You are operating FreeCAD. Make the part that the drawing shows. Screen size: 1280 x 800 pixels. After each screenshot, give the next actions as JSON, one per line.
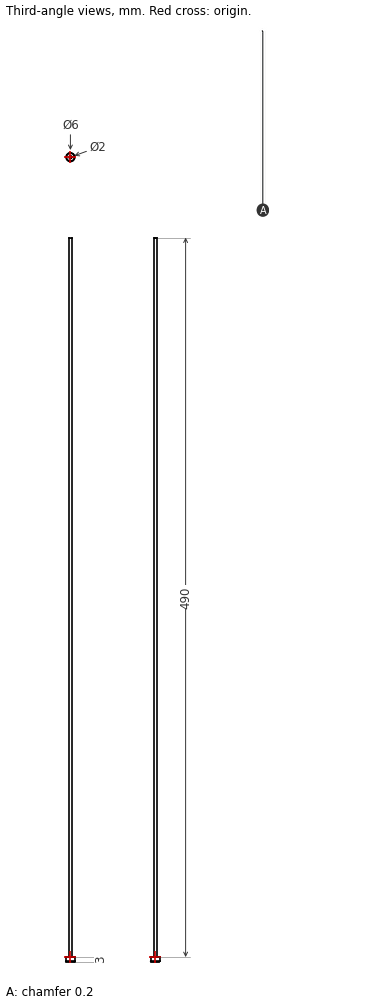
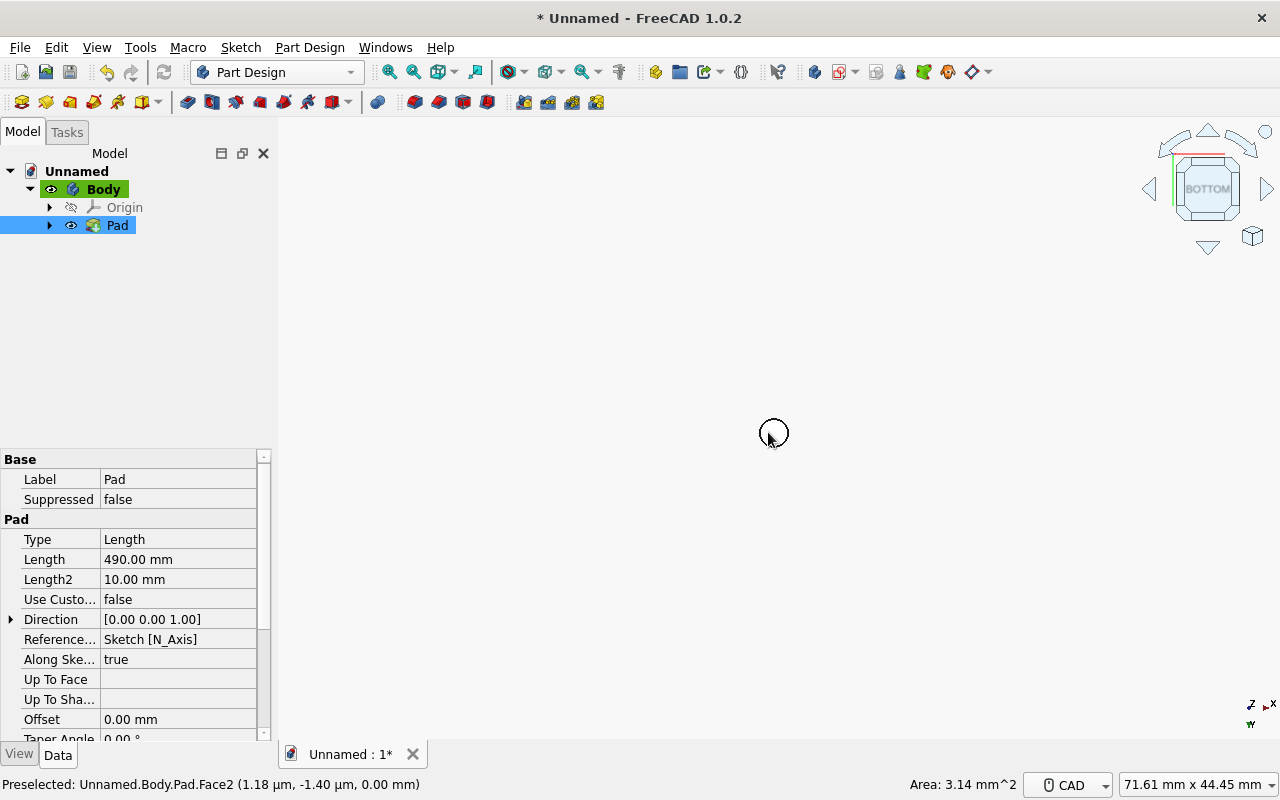
{"action": "left_click", "coordinate": [840, 72]}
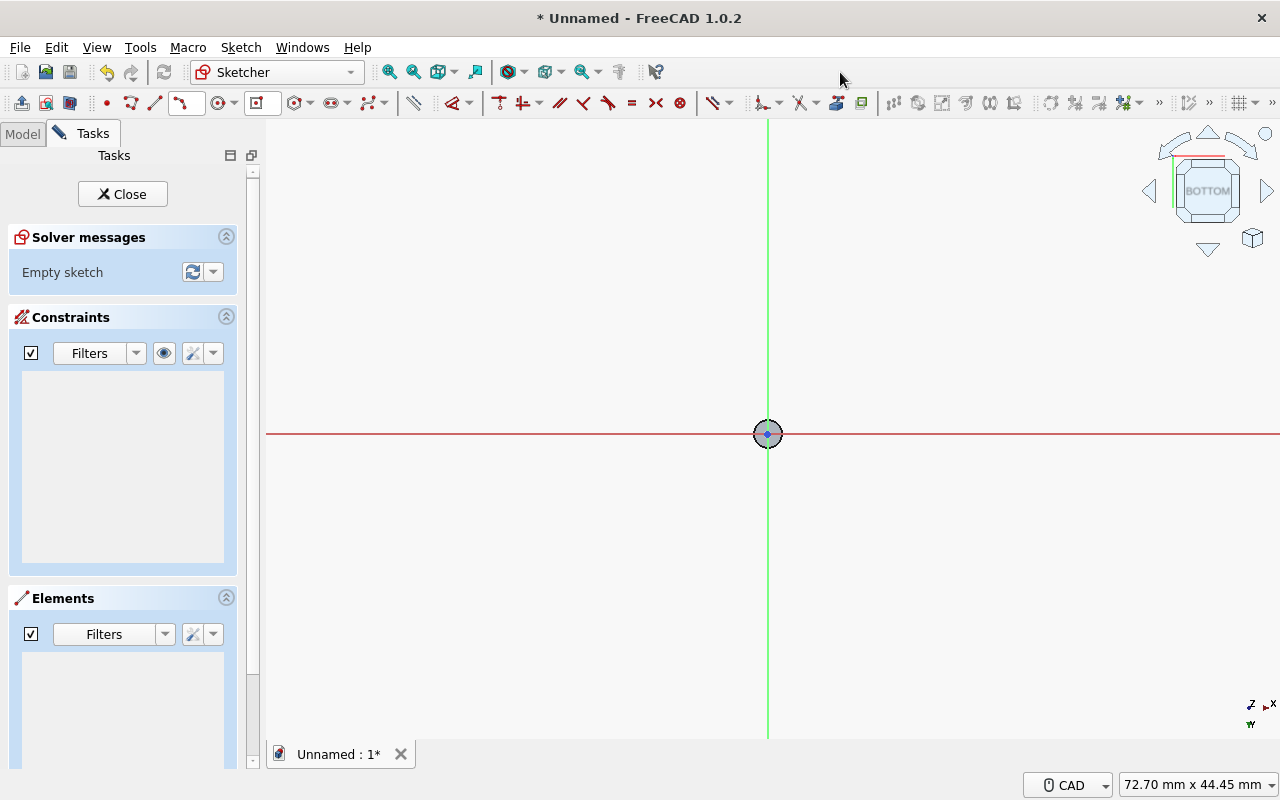
{"action": "scroll", "coordinate": [784, 435], "scroll_direction": "up", "scroll_amount": 8}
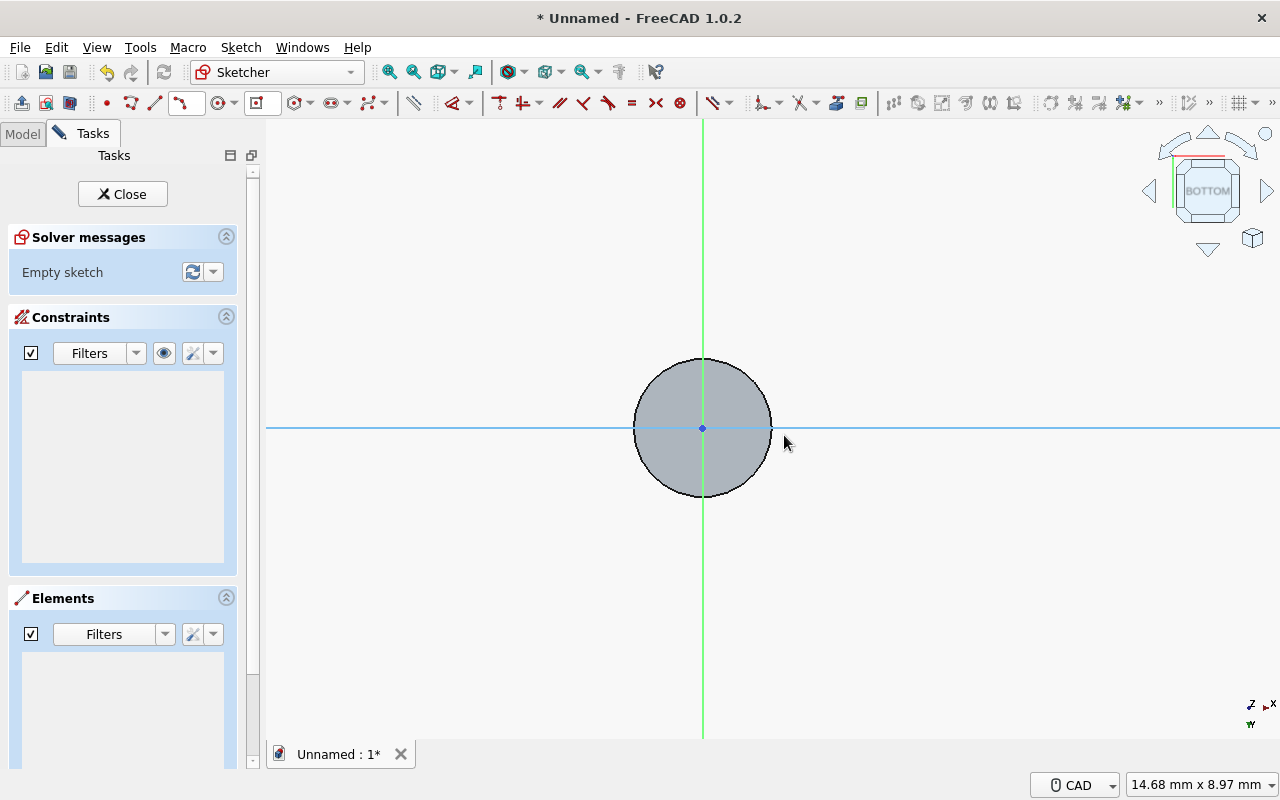
{"action": "key", "text": "g c"}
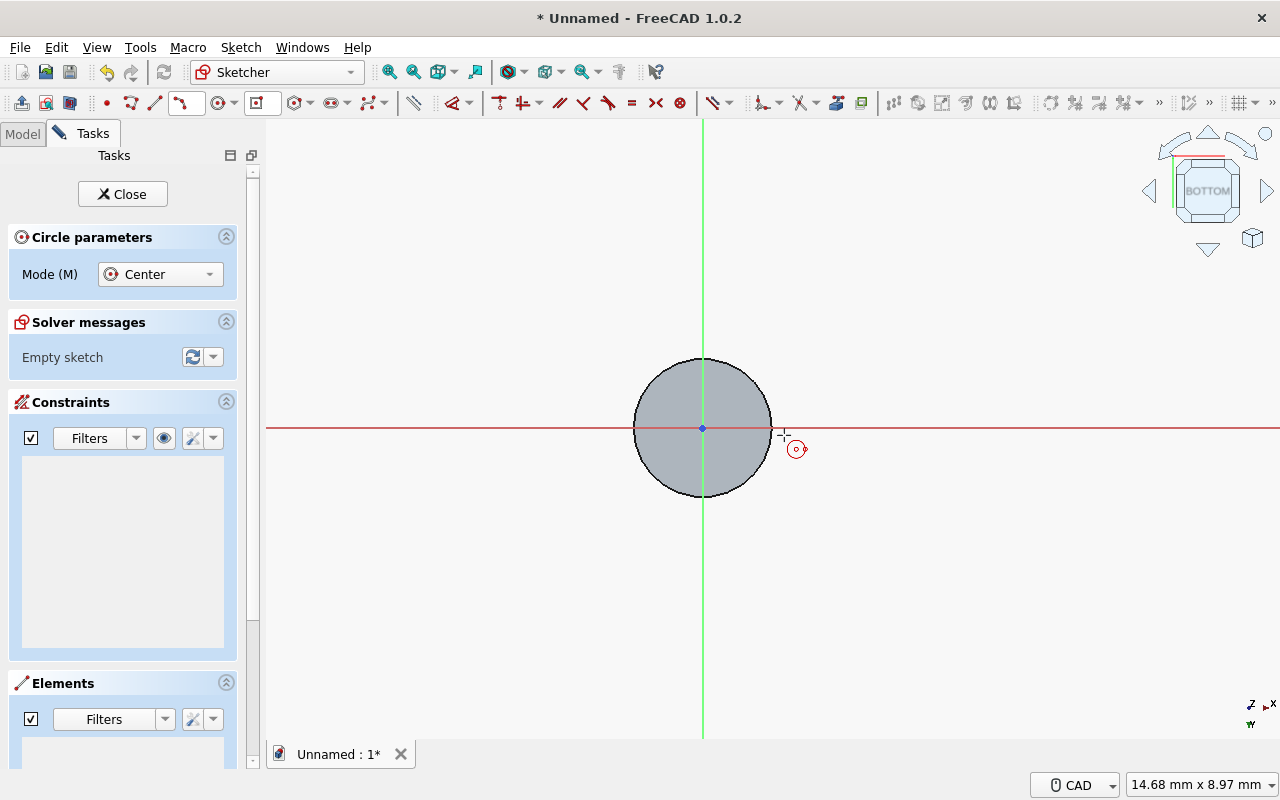
{"action": "left_click", "coordinate": [703, 428]}
{"action": "left_click", "coordinate": [849, 282]}
{"action": "key", "text": "Escape"}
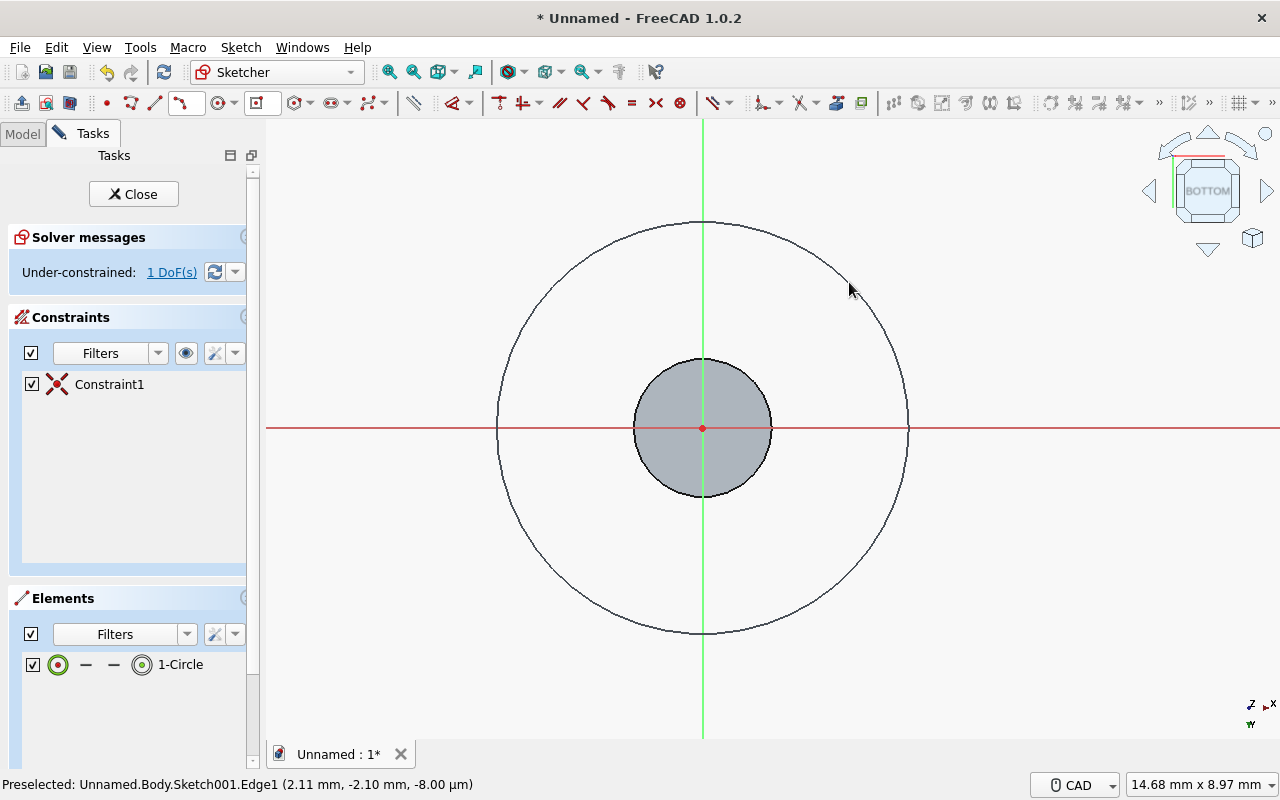
{"action": "key", "text": "d"}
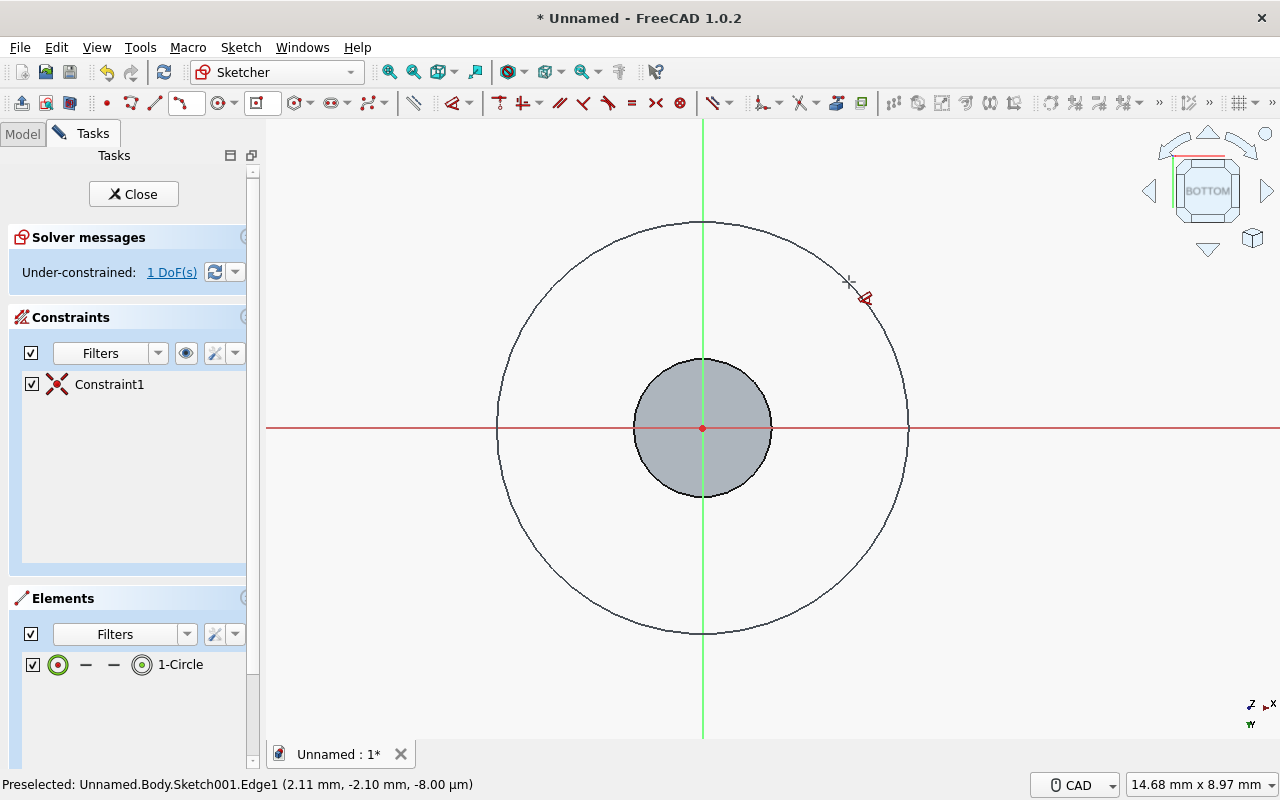
{"action": "left_click", "coordinate": [848, 282]}
{"action": "left_click", "coordinate": [871, 259]}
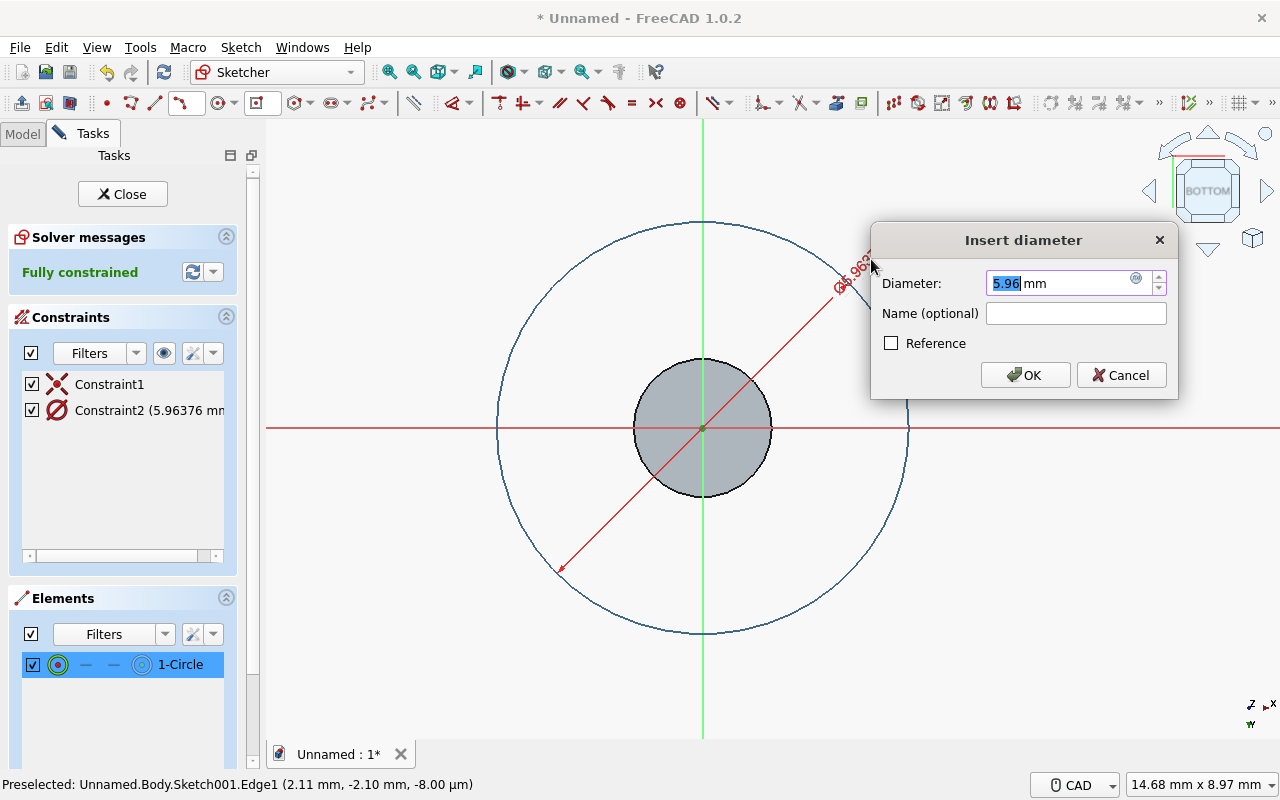
{"action": "type", "text": "6"}
{"action": "key", "text": "Return"}
{"action": "key", "text": "Escape"}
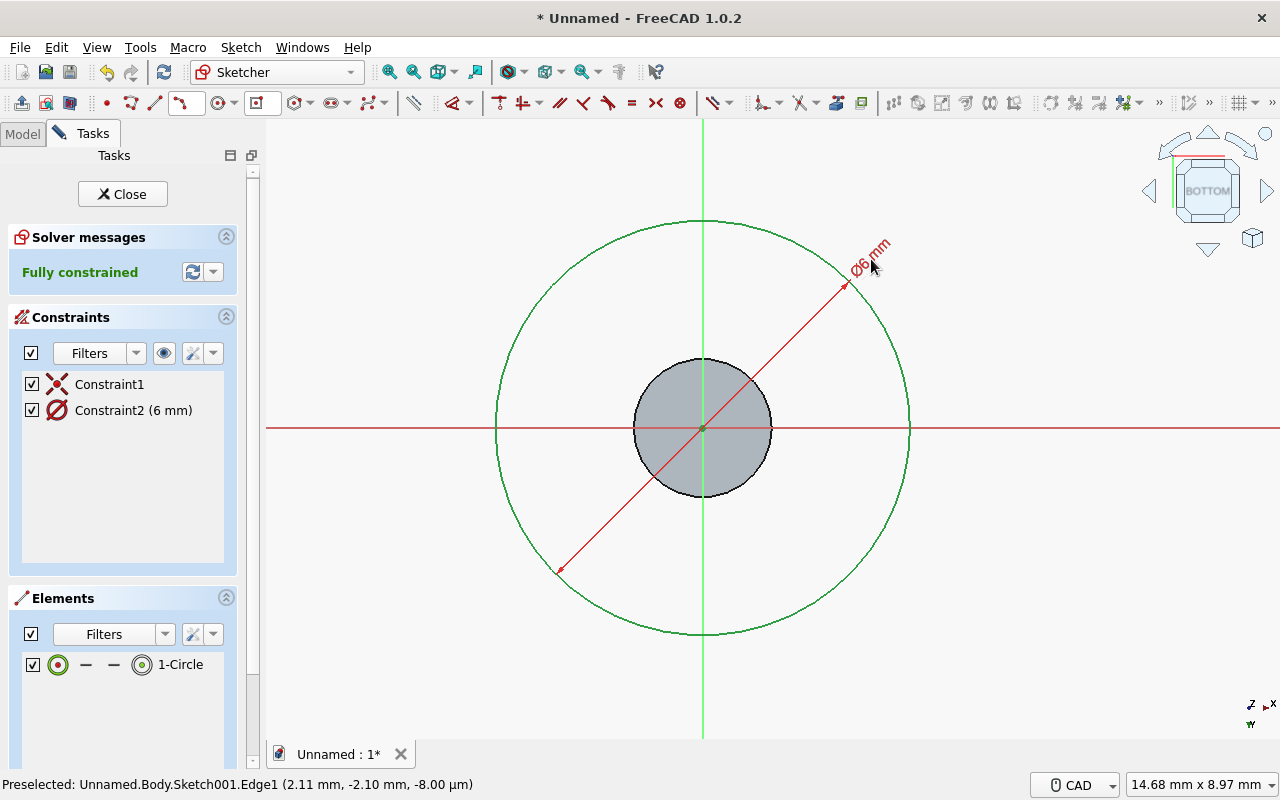
{"action": "left_click", "coordinate": [123, 194]}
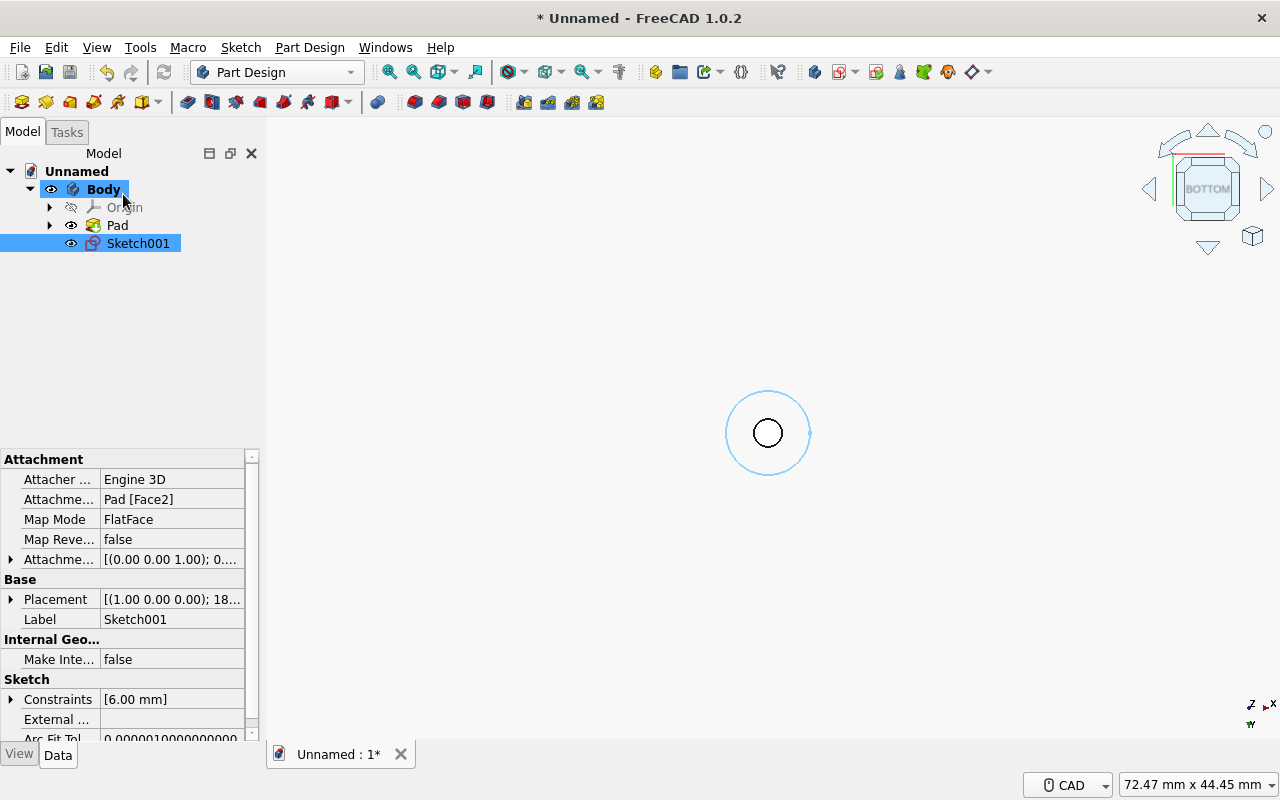
{"action": "left_click", "coordinate": [22, 102]}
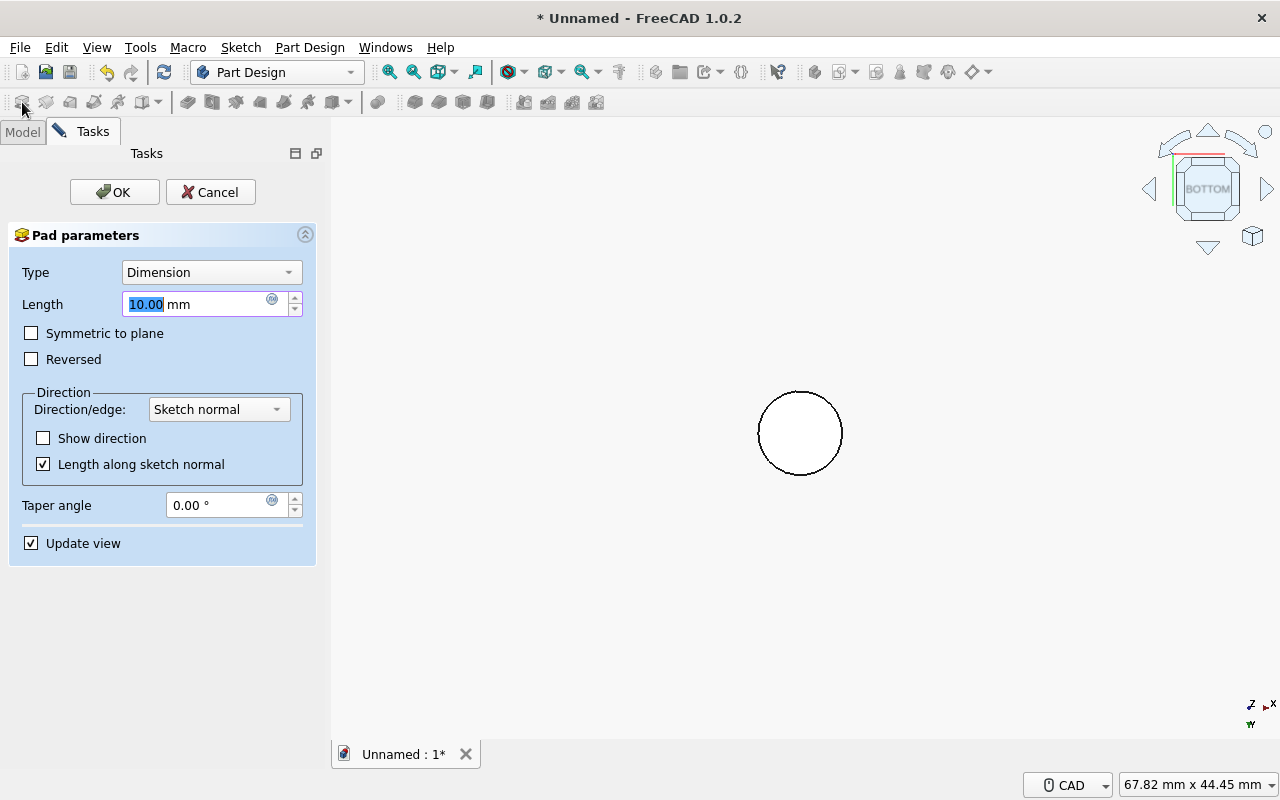
{"action": "type", "text": "3"}
{"action": "key", "text": "Tab"}